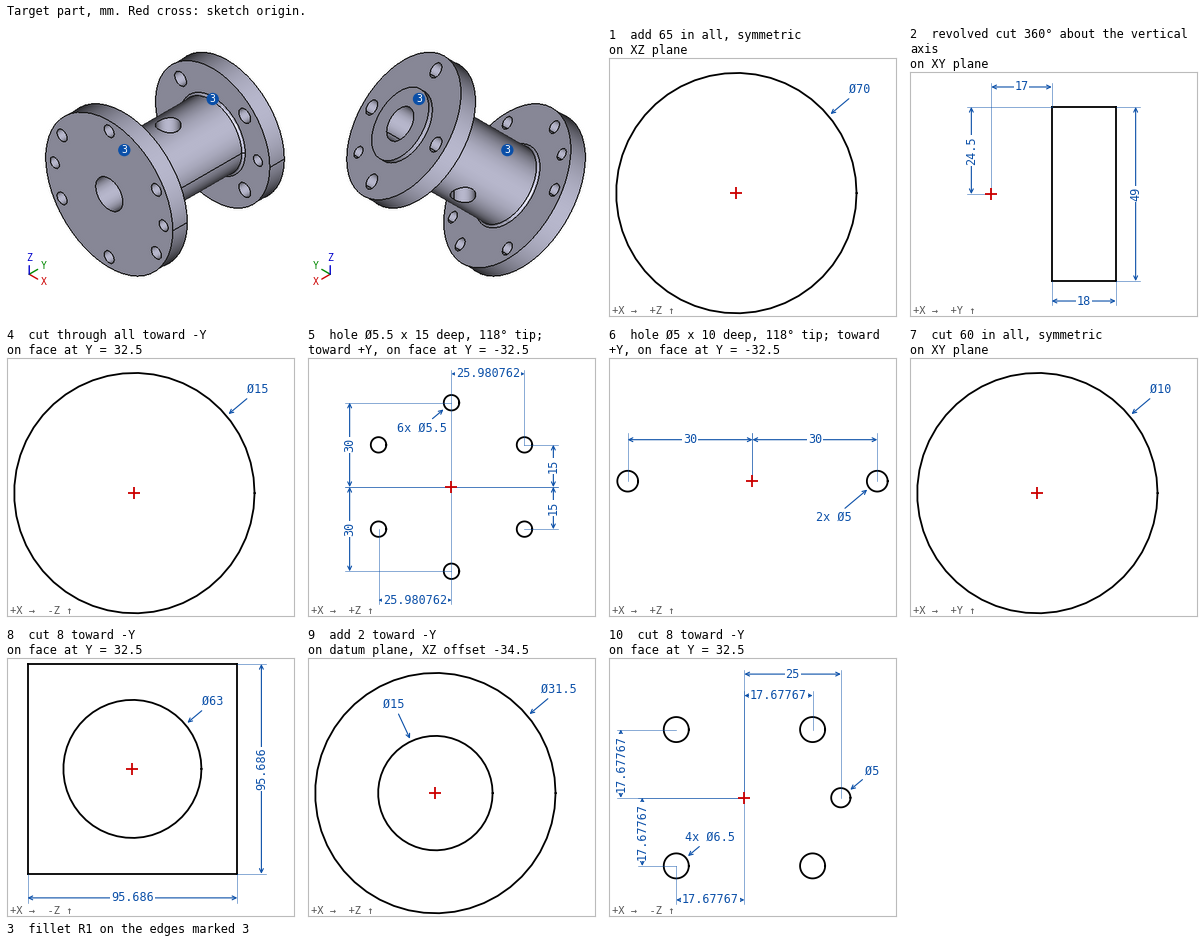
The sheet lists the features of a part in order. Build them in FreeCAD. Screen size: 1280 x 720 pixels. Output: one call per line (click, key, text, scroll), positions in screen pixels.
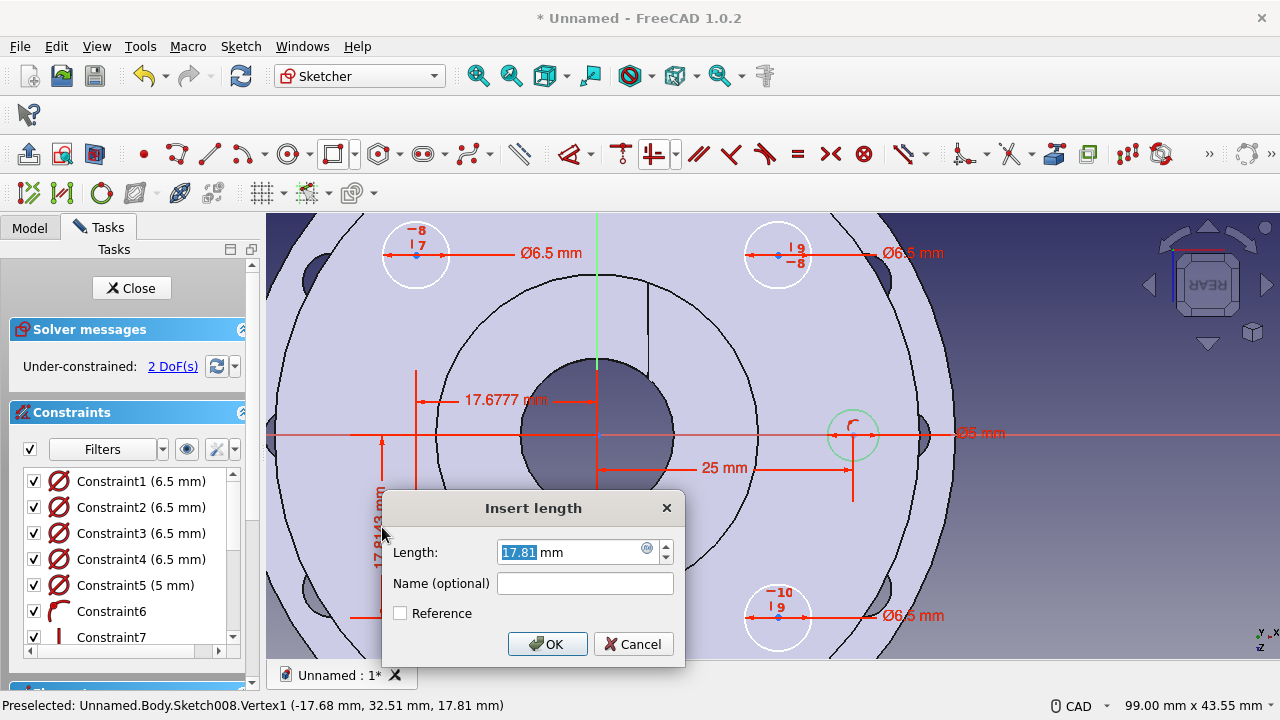
text(17.67767)
key(Return)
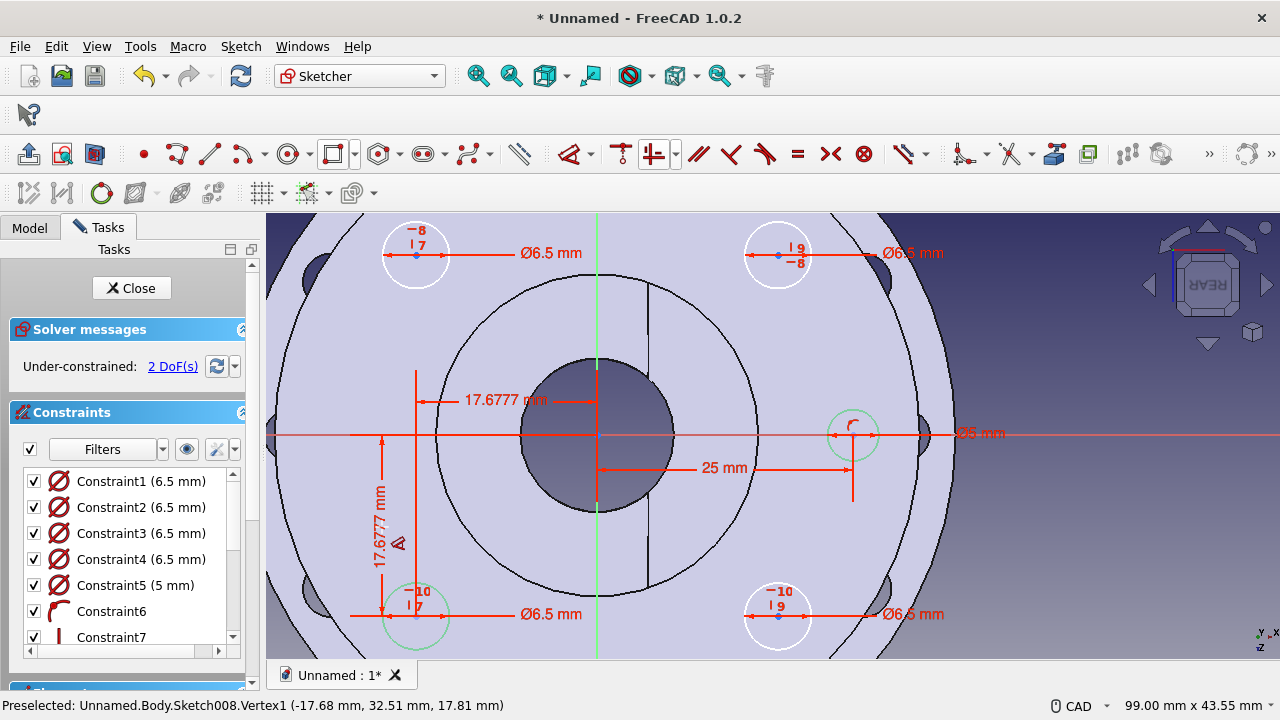
click(416, 255)
click(382, 345)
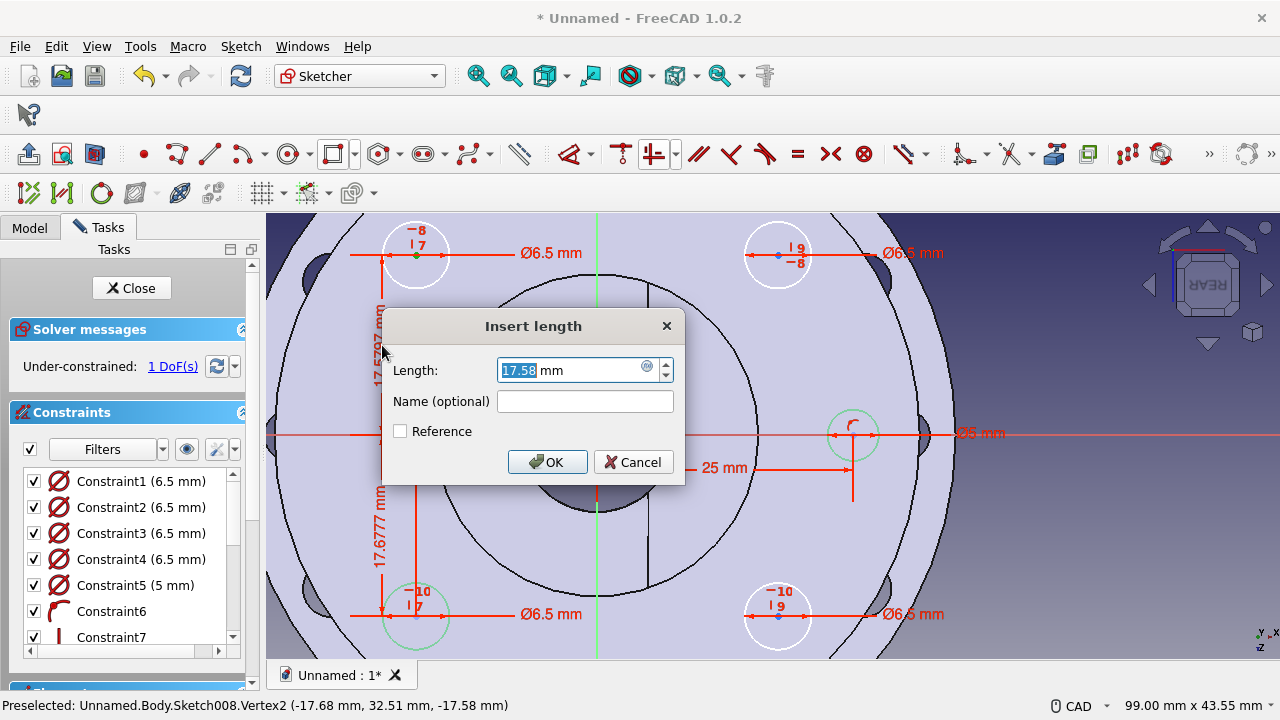
text(17.67767)
key(Return)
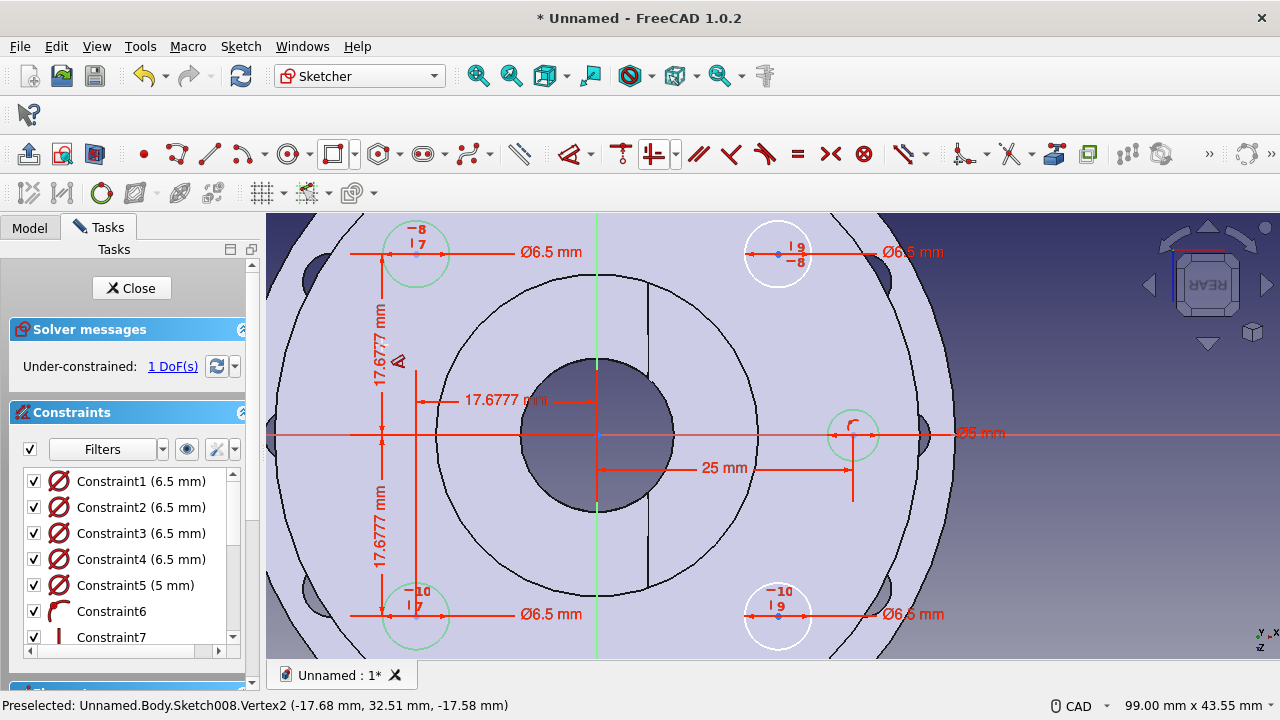
click(778, 254)
click(646, 469)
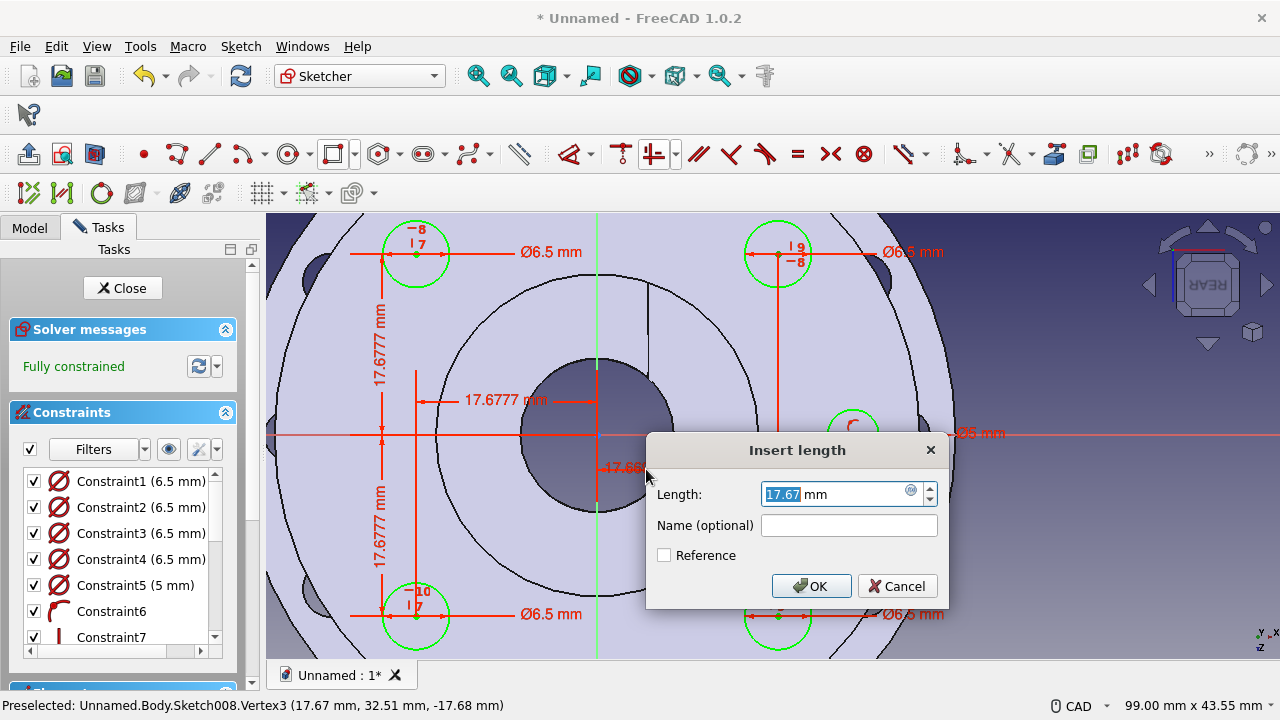
text(17.67767)
key(Return)
key(Escape)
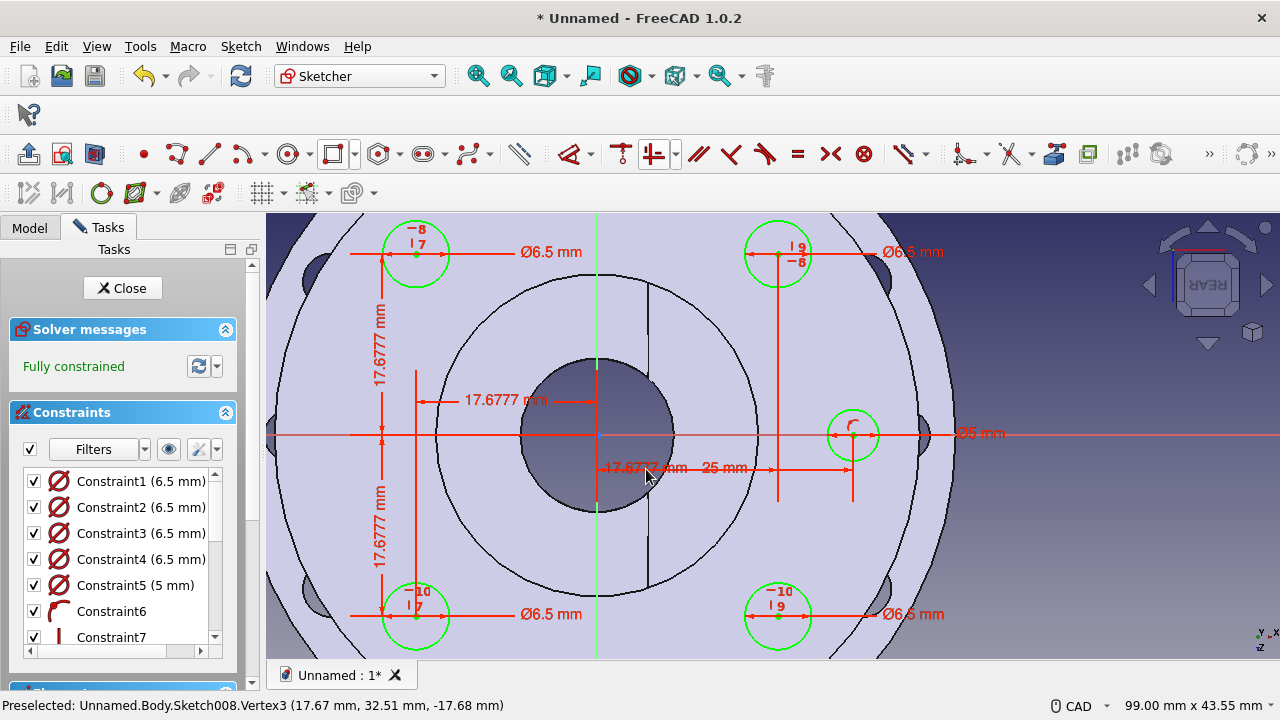
click(123, 288)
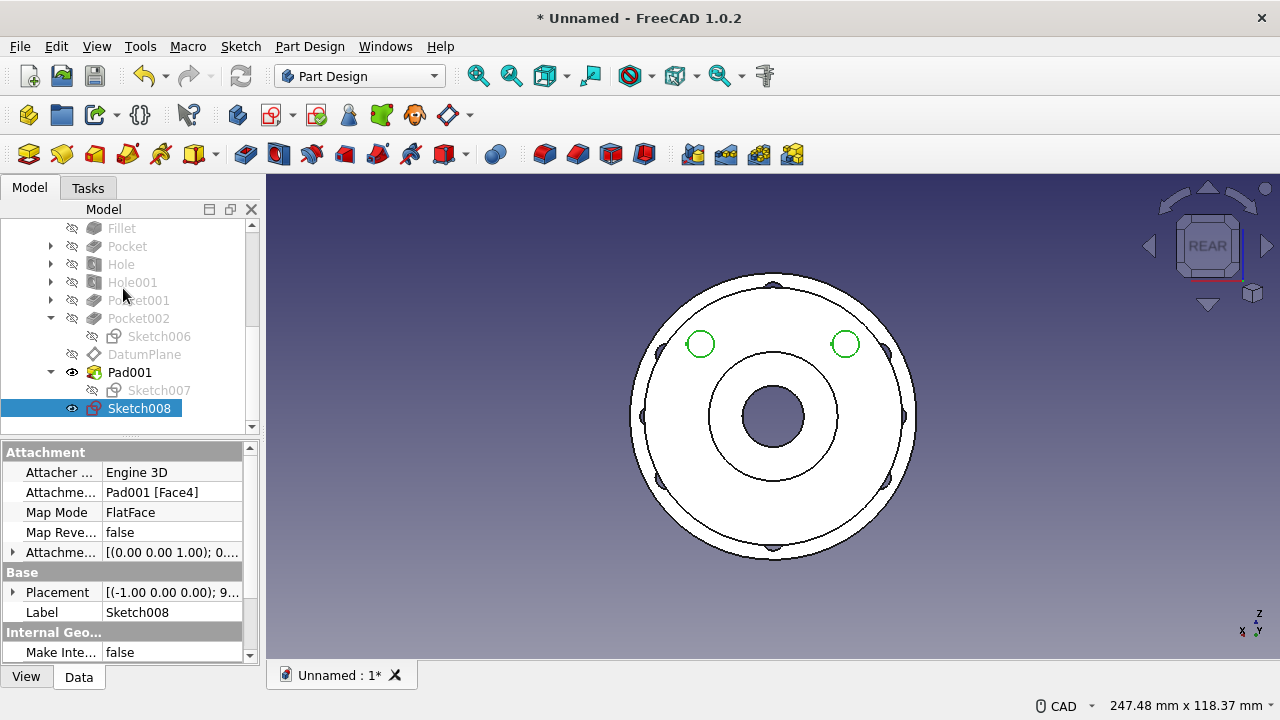
click(246, 154)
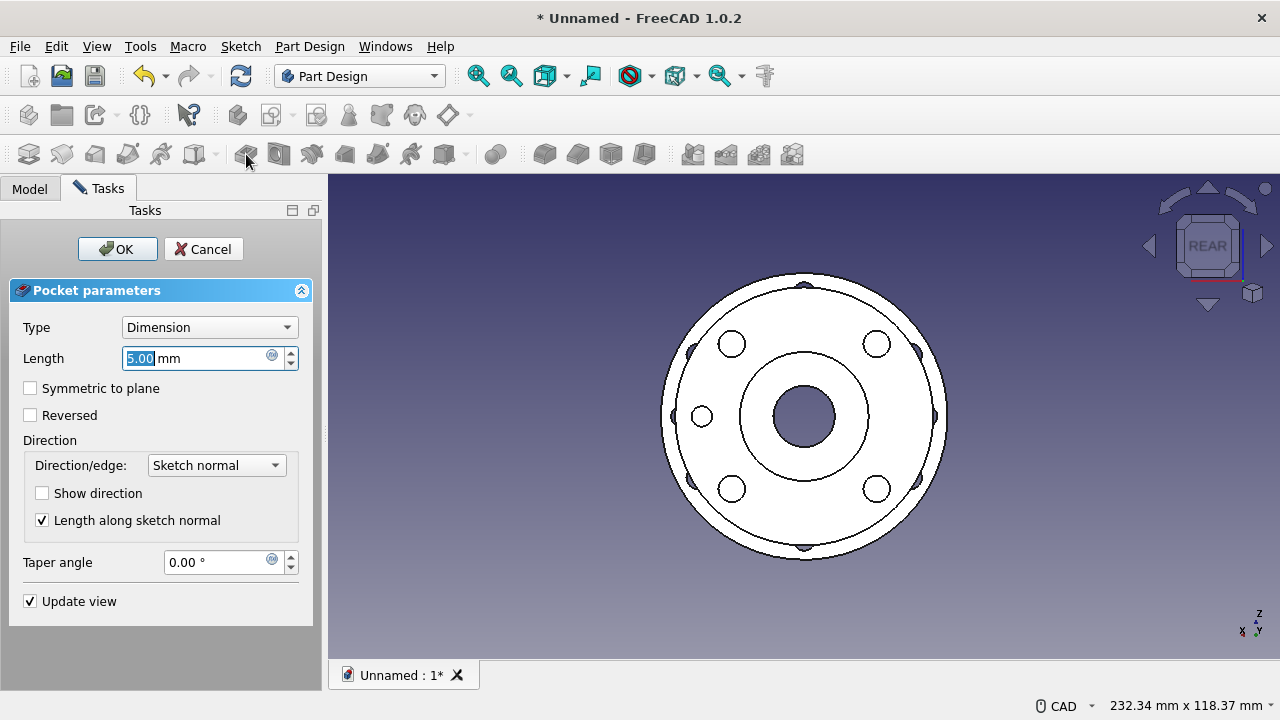
text(8)
key(Tab)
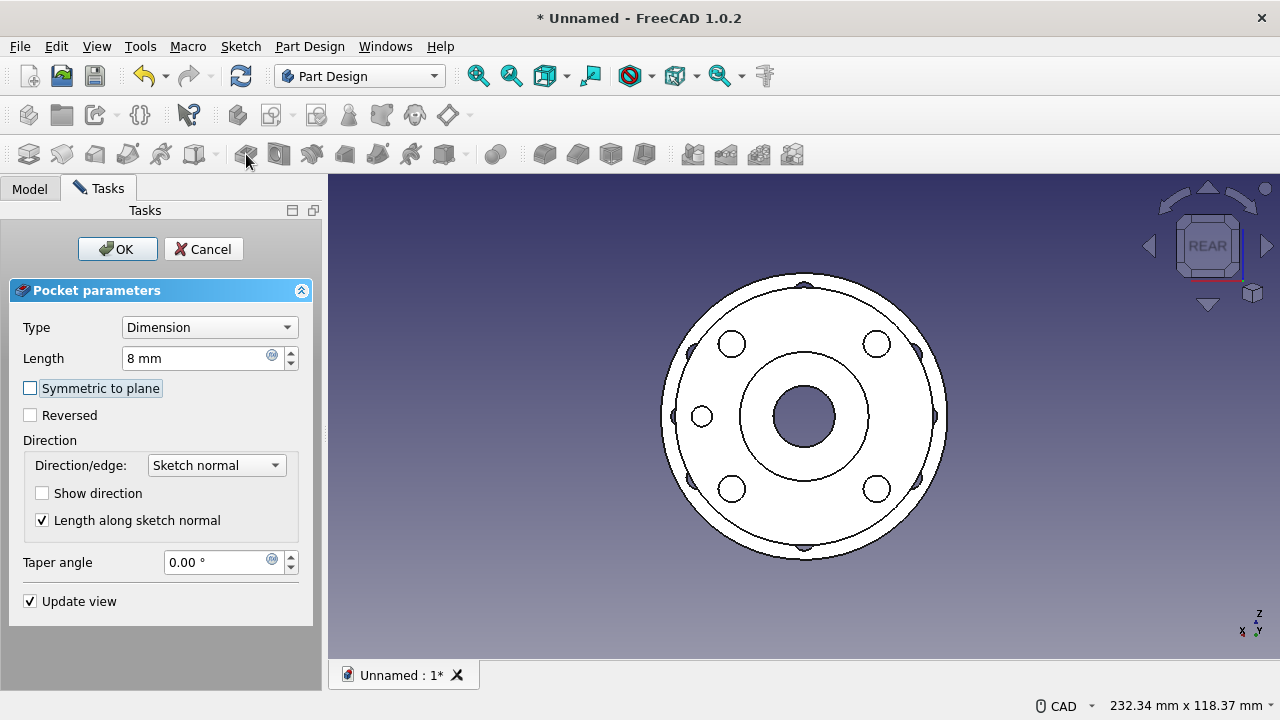
click(118, 249)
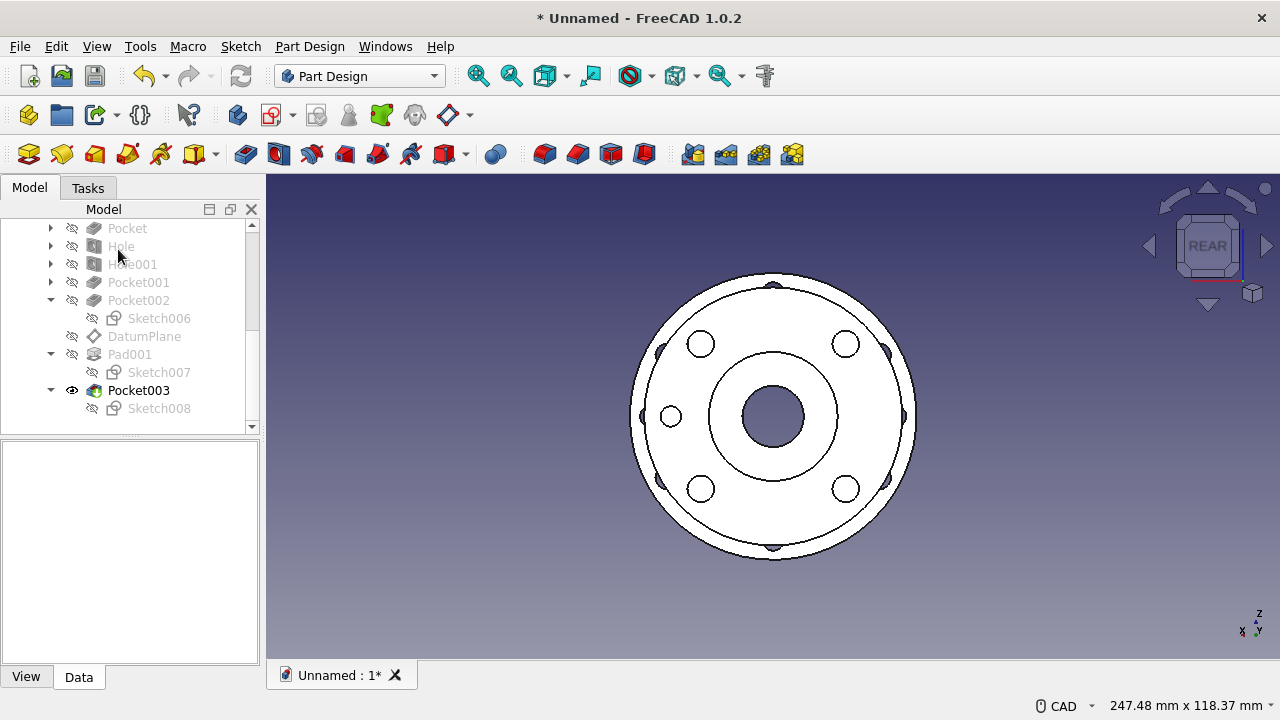
key(0)